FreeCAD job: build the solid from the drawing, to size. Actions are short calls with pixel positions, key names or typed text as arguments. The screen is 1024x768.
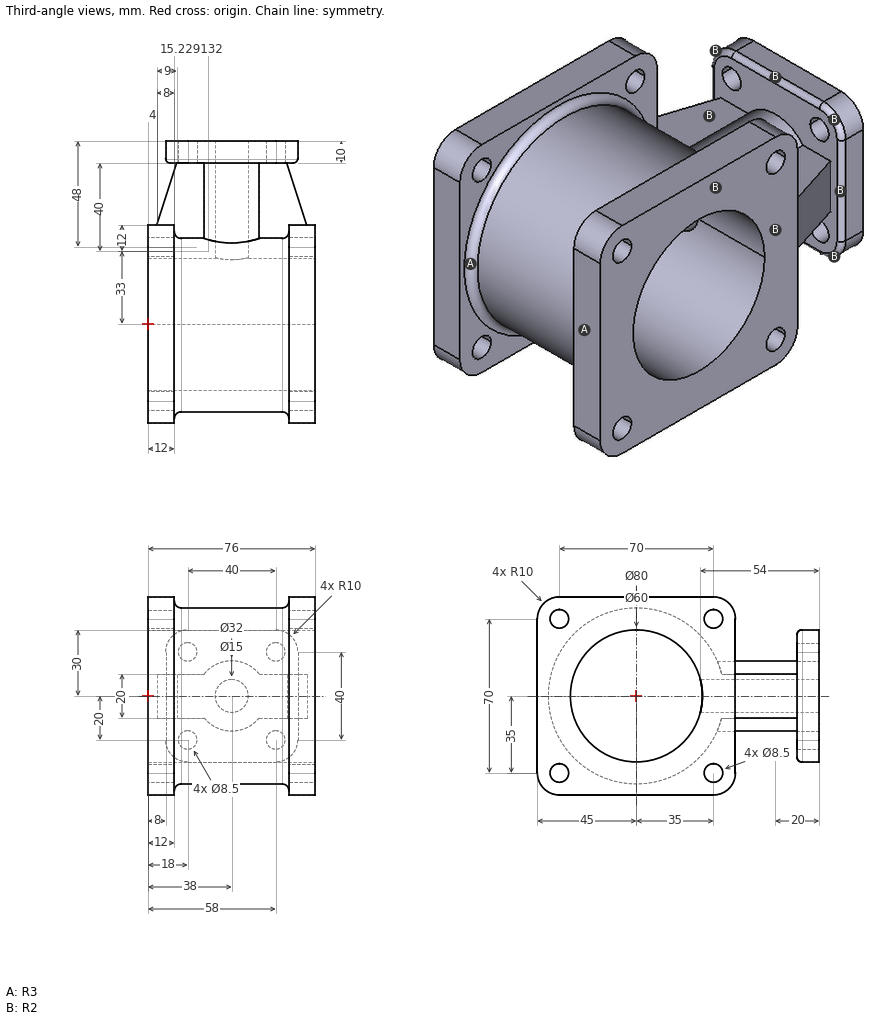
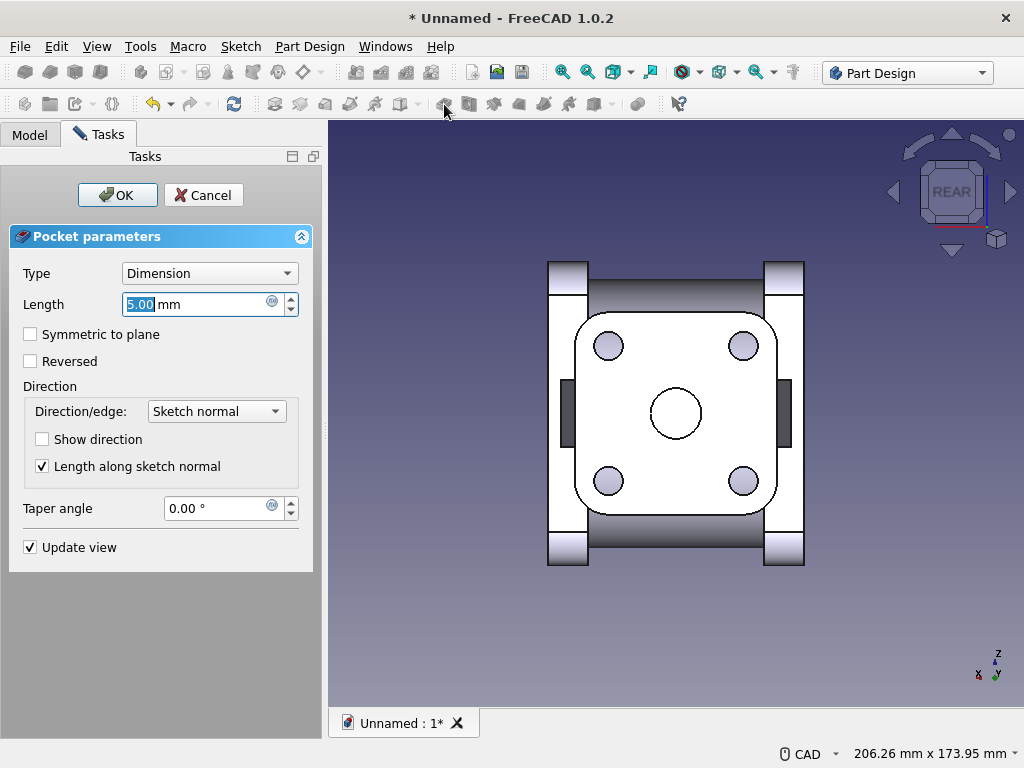
text(54)
key(Tab)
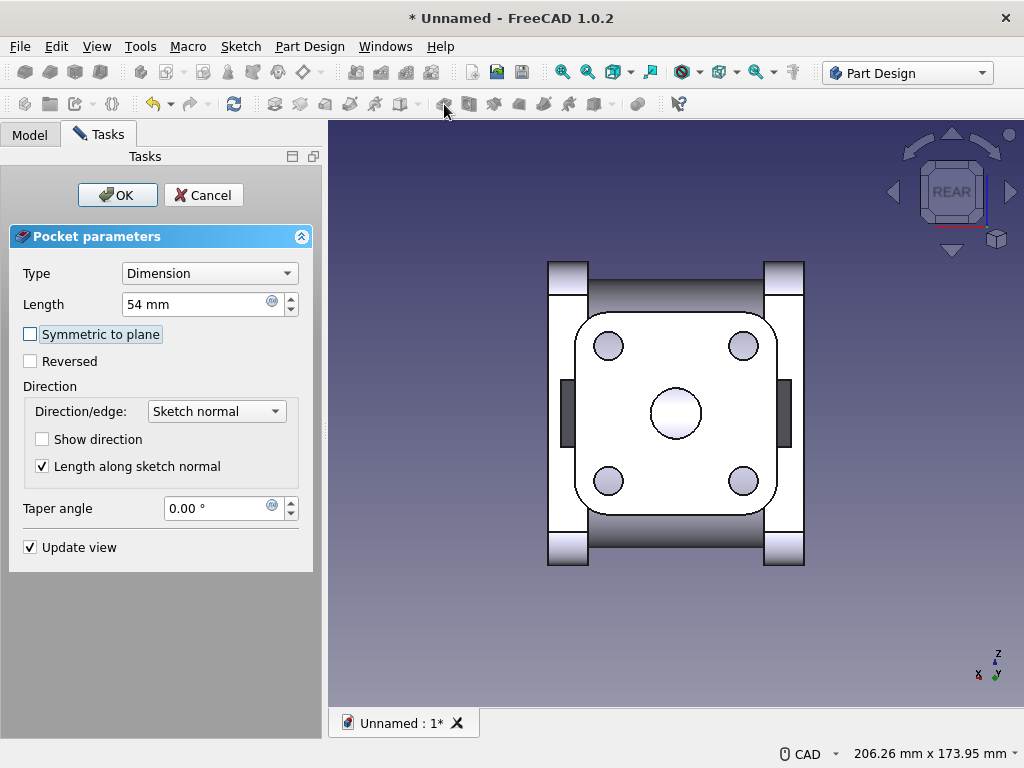
click(118, 195)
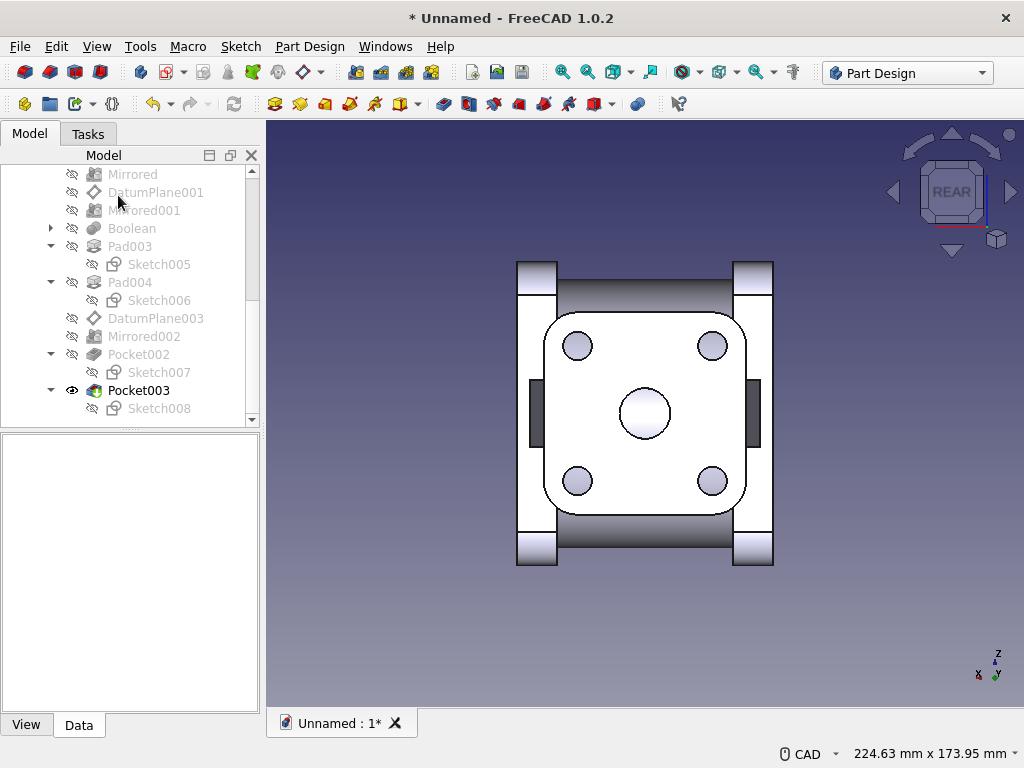
key(0)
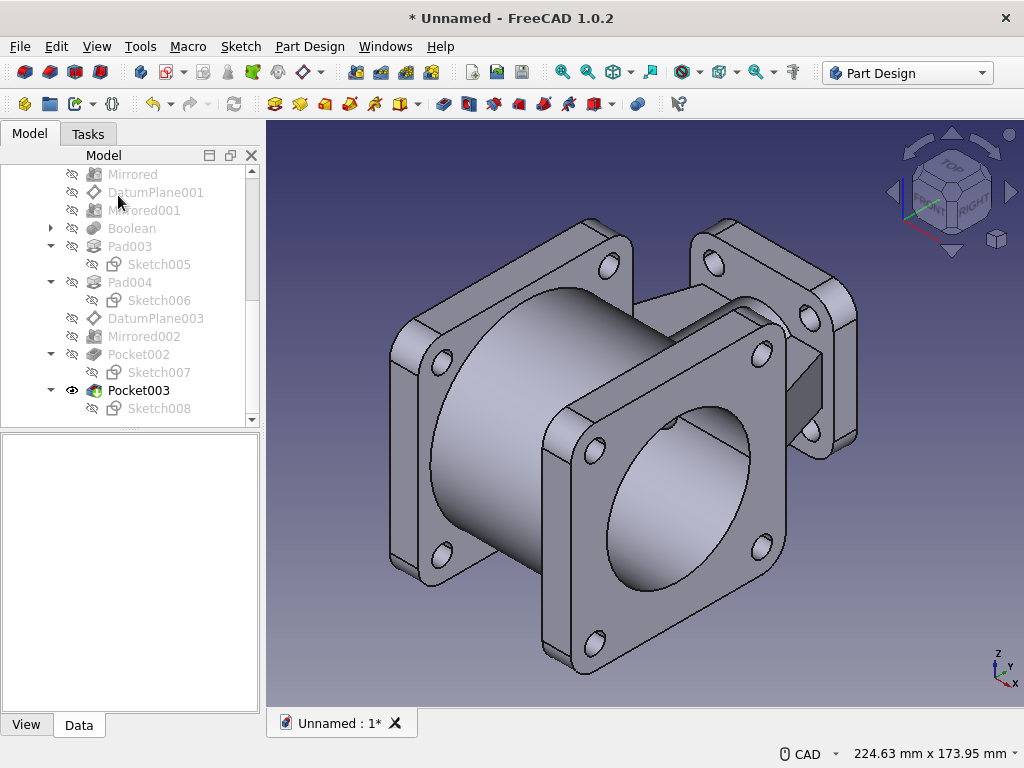
key(2)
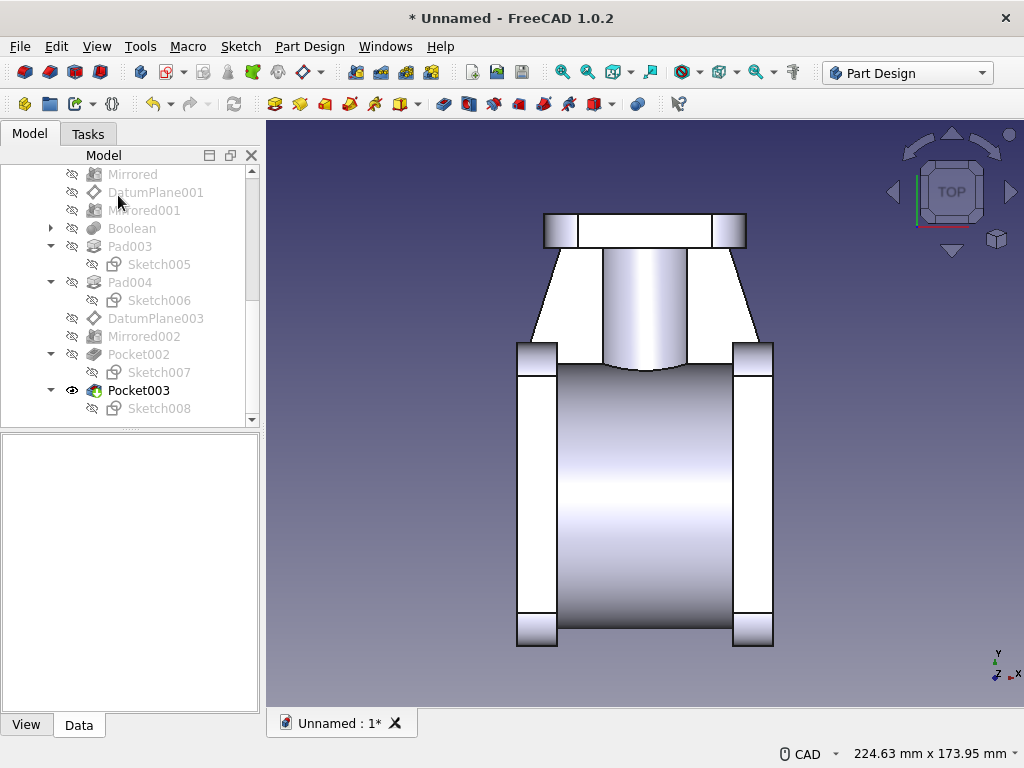
key(1)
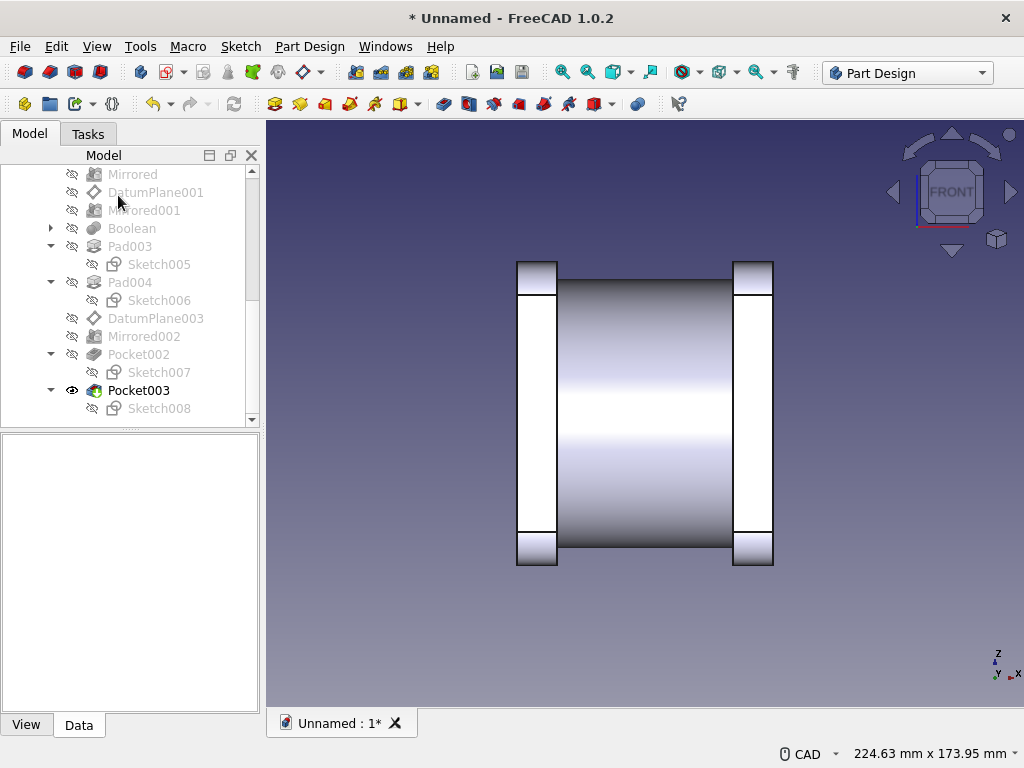
key(3)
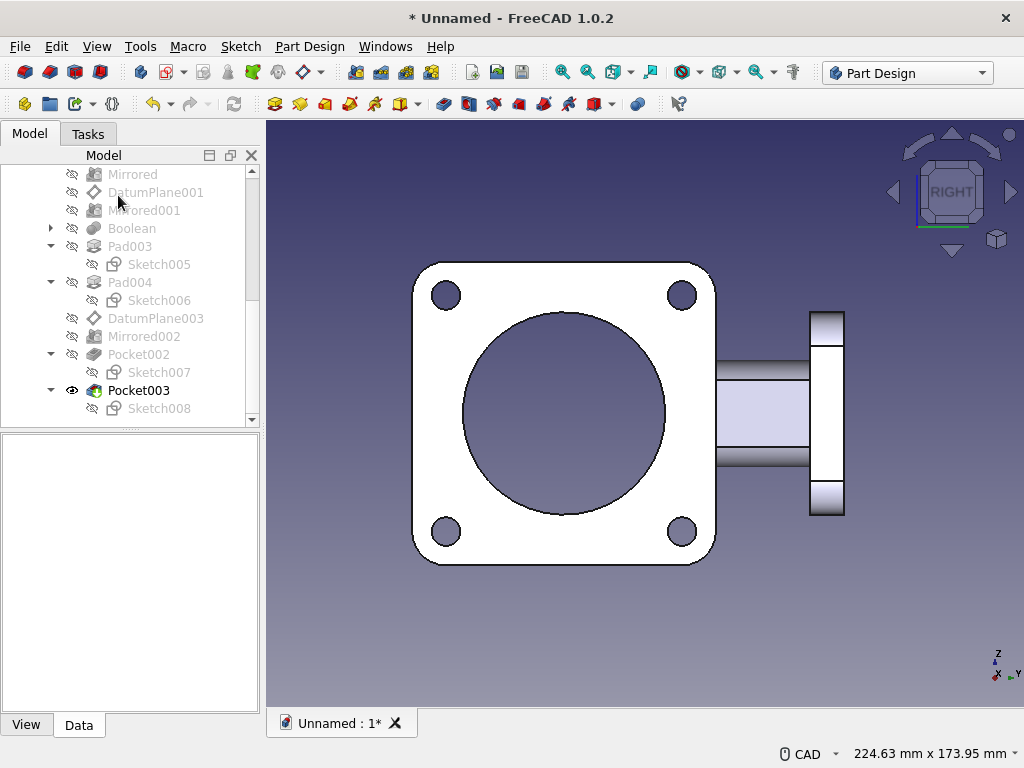
key(5)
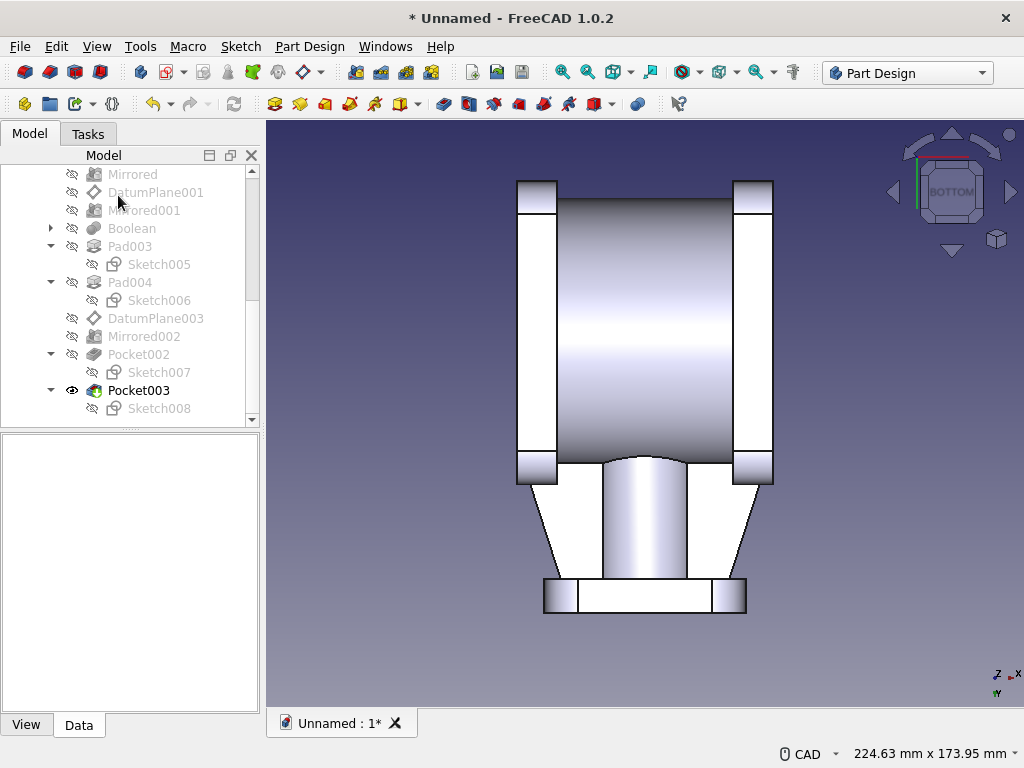
key(4)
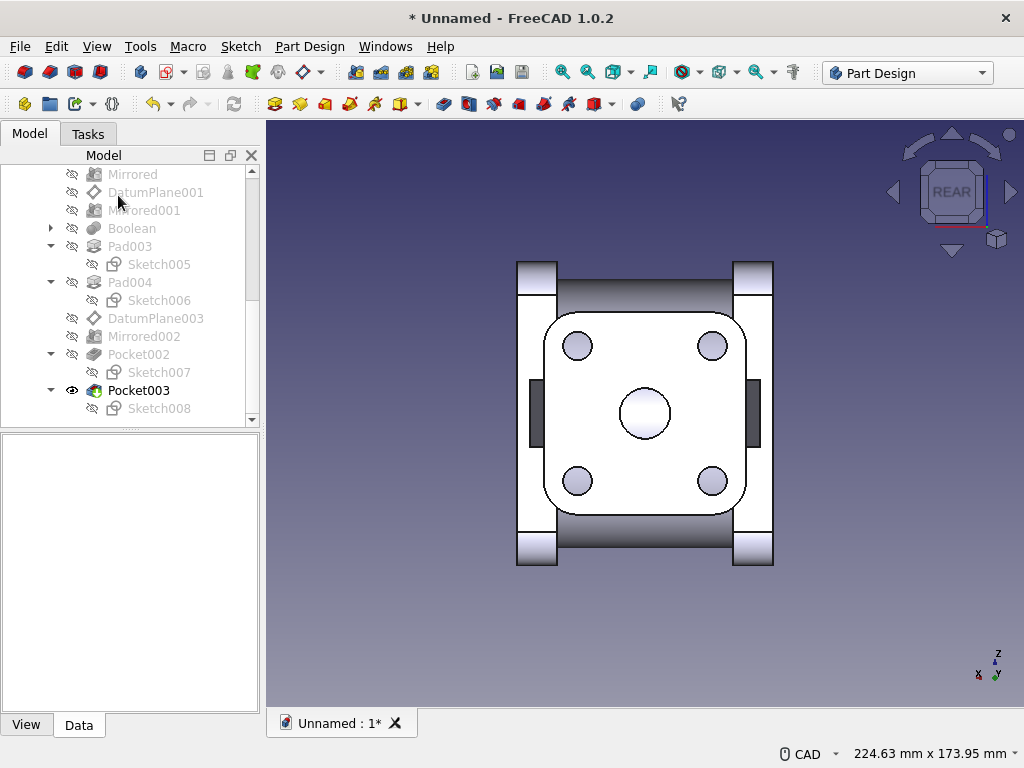
key(6)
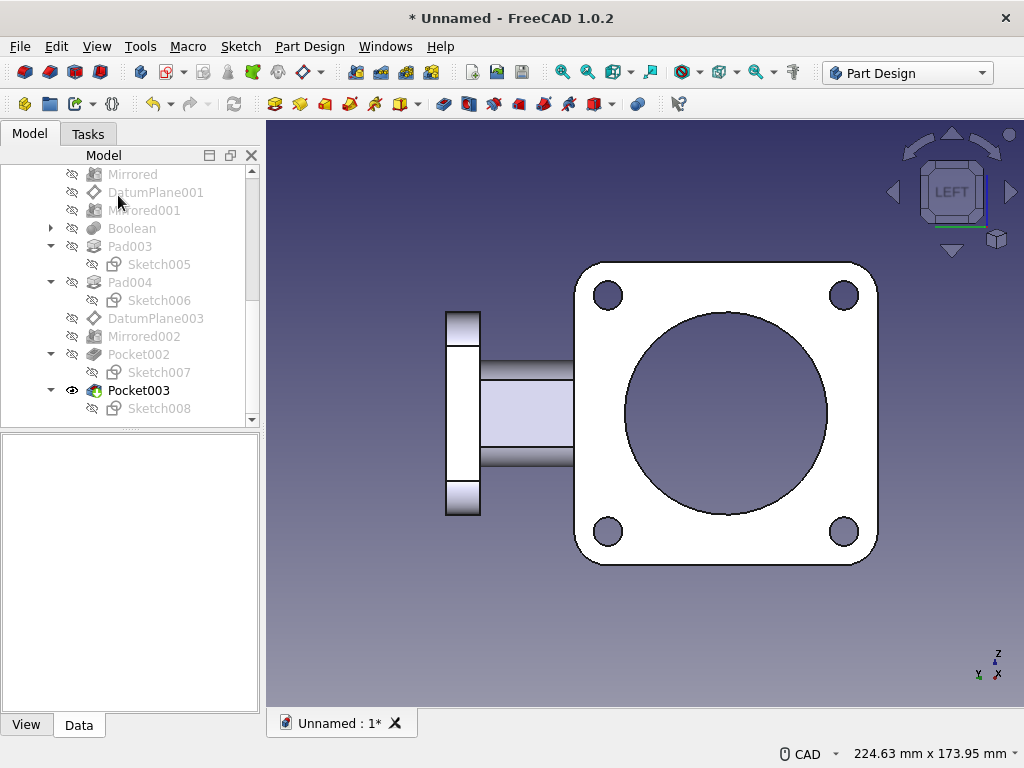
key(v)
key(3)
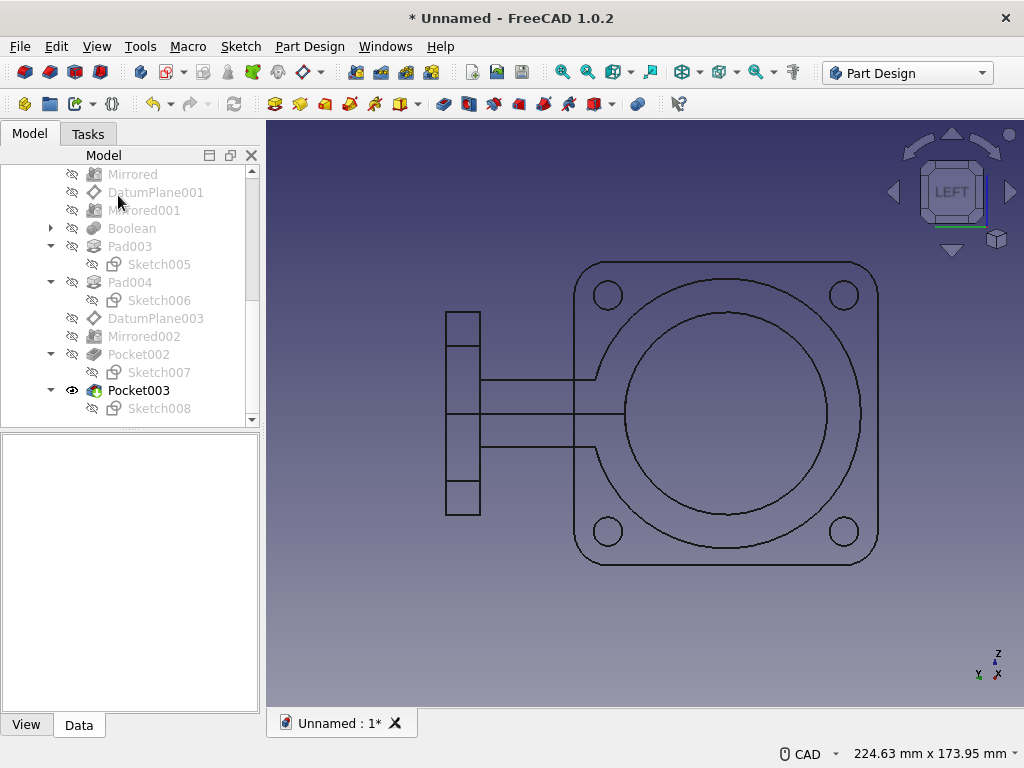
key(0)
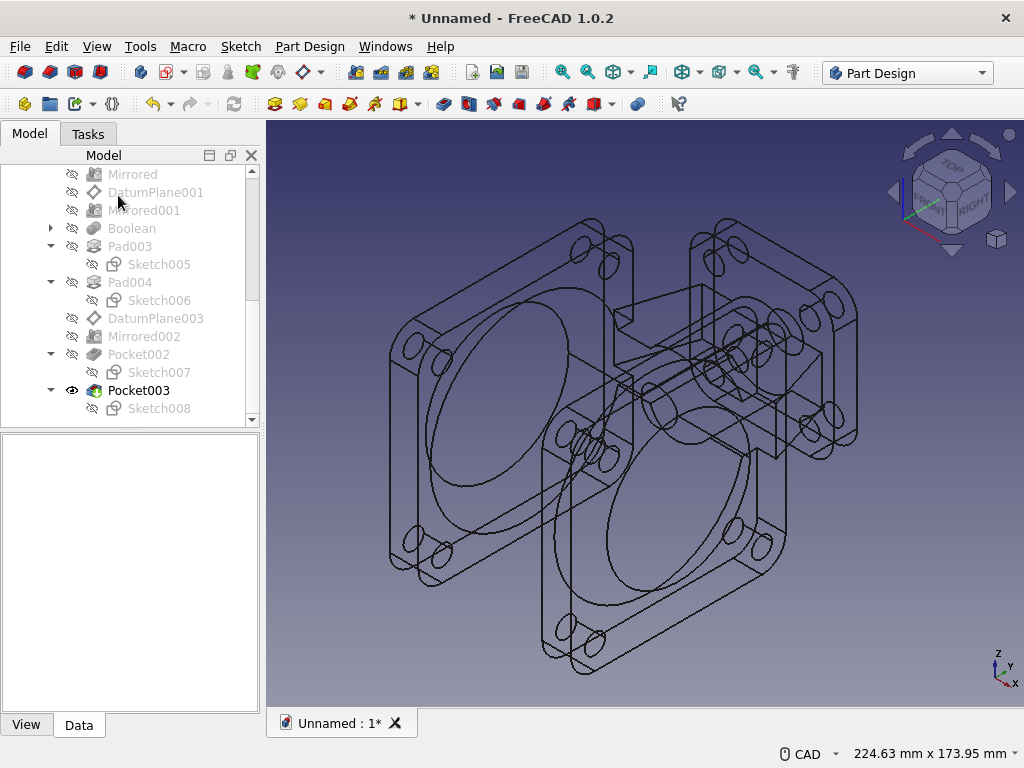
click(430, 465)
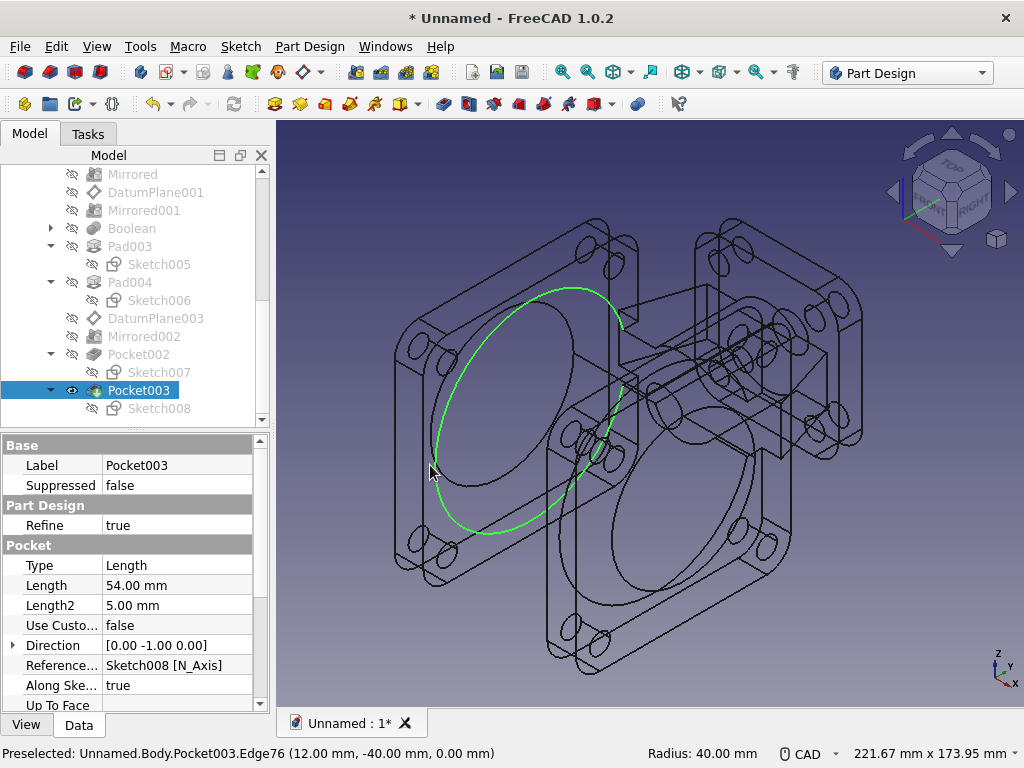
click(559, 536, ctrl)